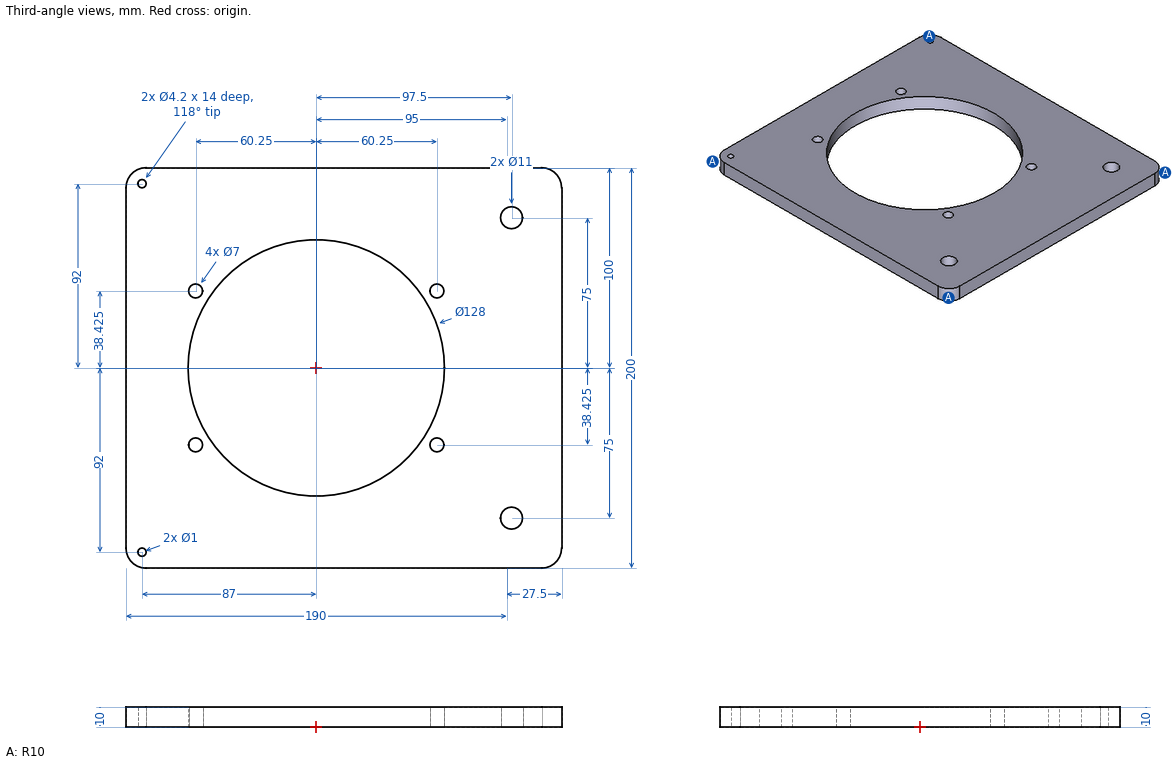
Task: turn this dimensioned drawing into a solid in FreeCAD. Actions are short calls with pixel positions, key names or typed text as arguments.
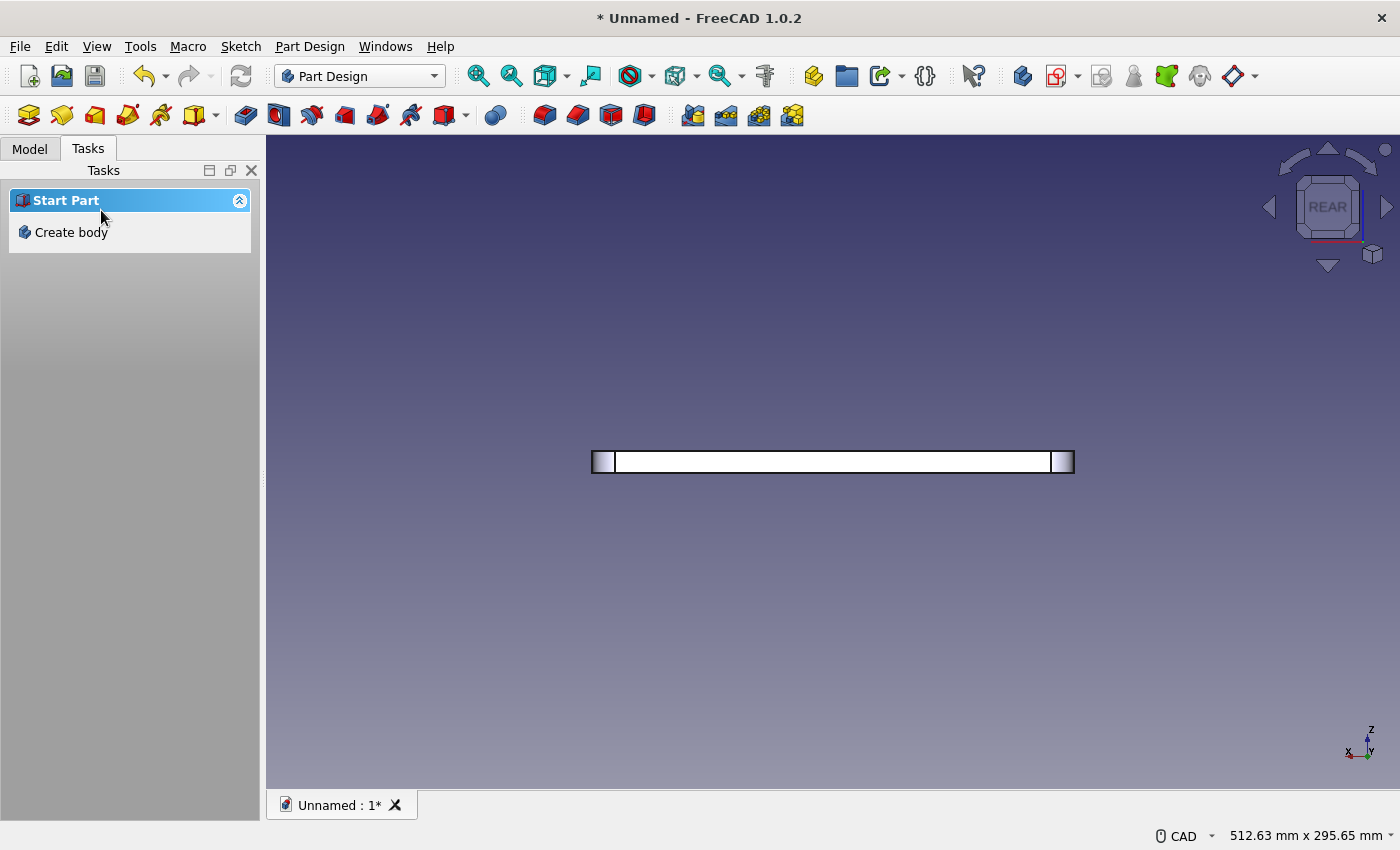
key(0)